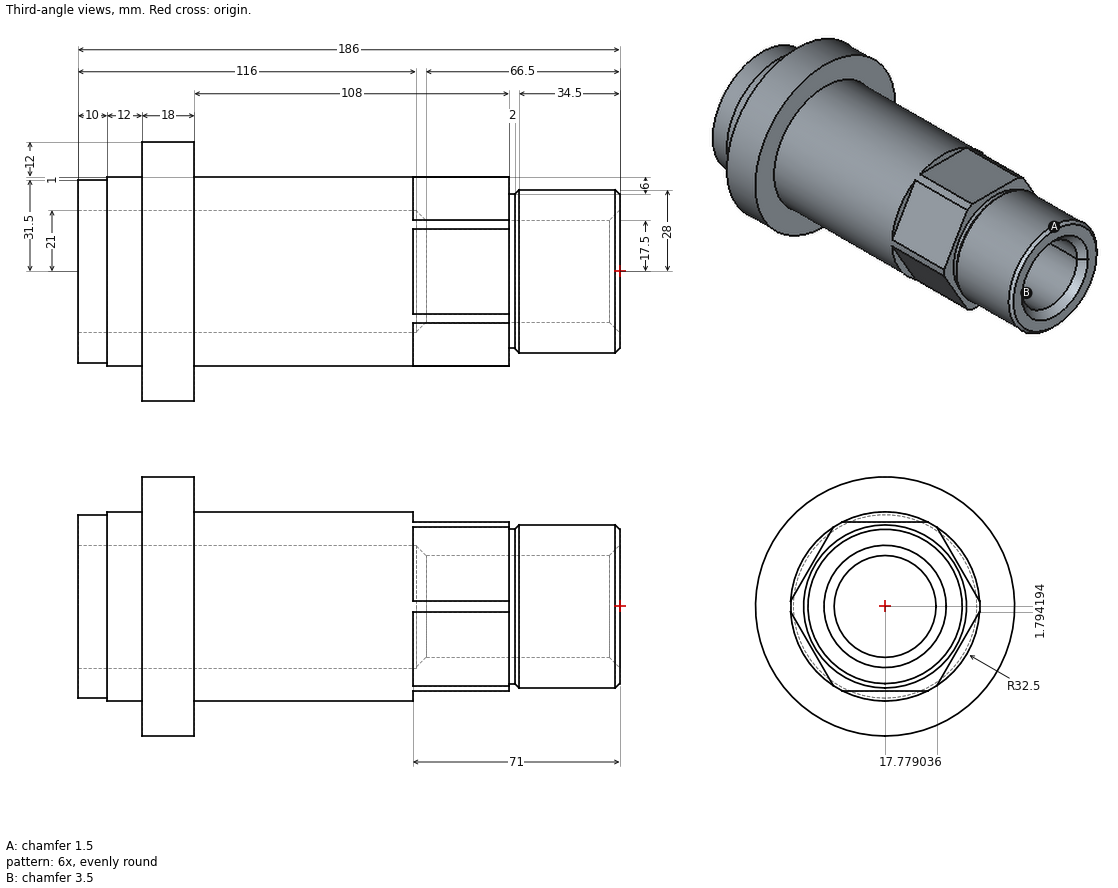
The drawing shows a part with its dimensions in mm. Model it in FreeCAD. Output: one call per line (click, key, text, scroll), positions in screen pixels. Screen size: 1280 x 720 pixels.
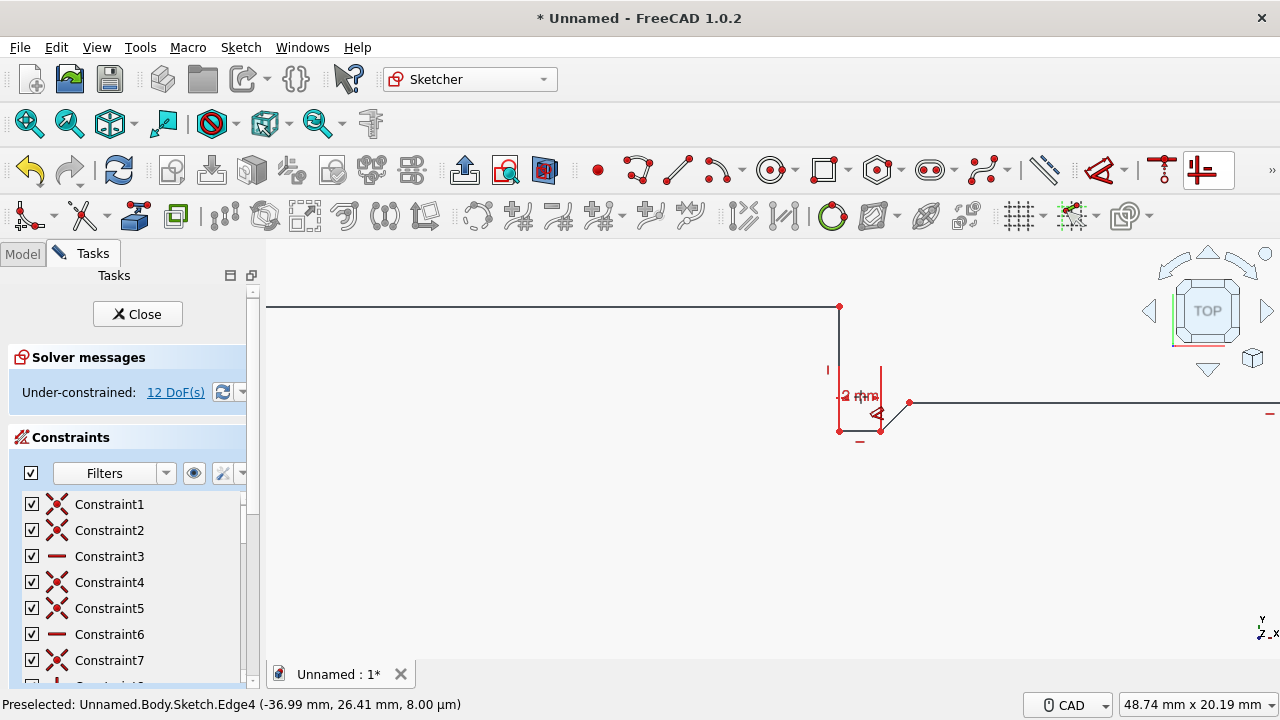
click(839, 394)
click(873, 369)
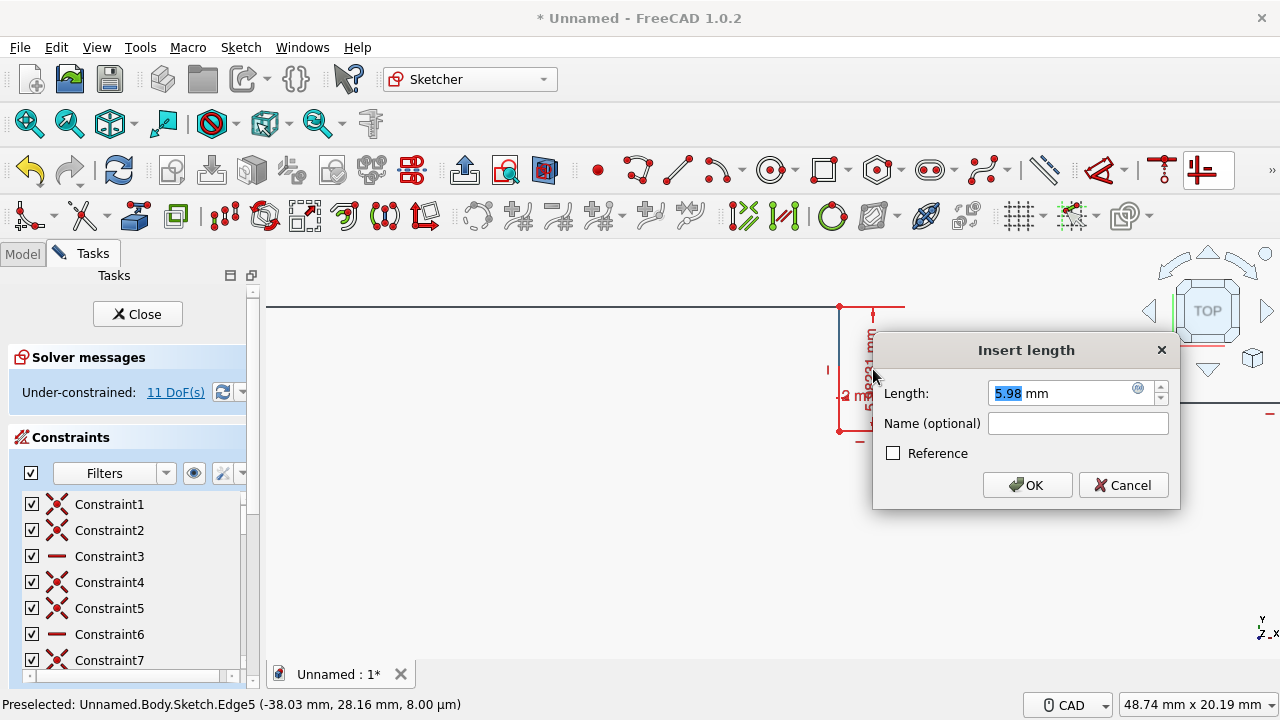
text(6)
key(Return)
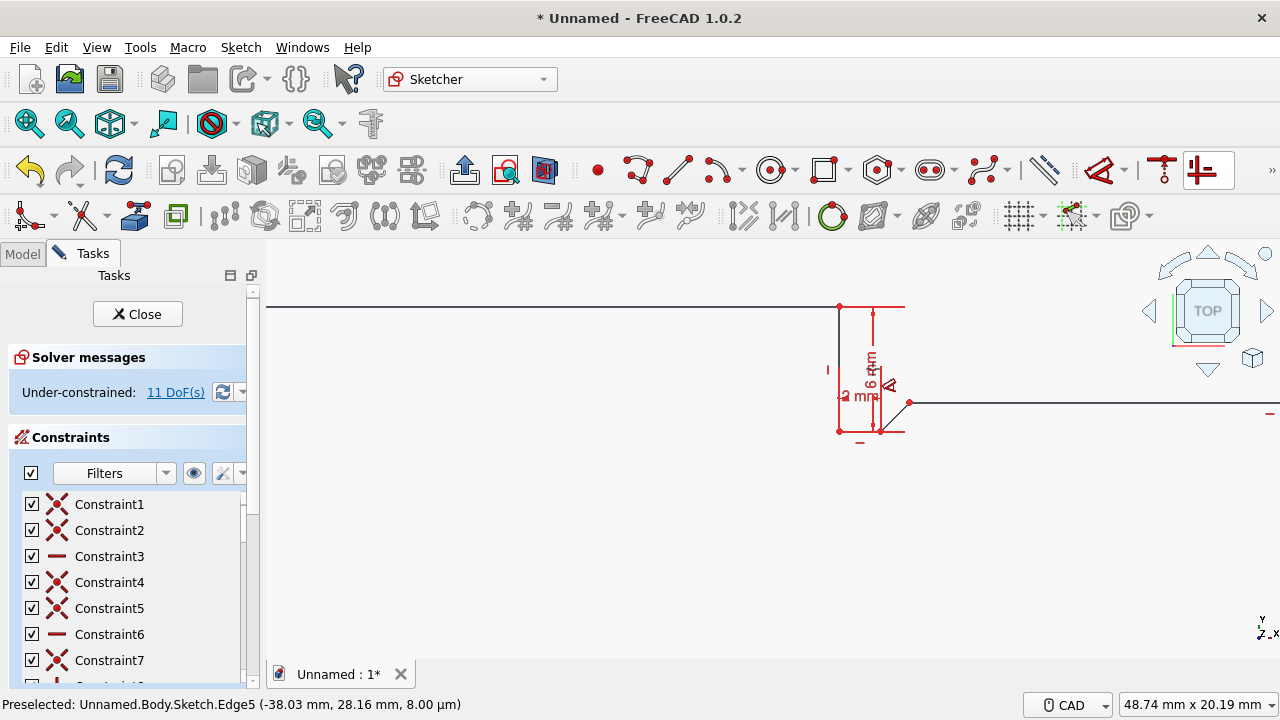
scroll(904, 435, down, 9)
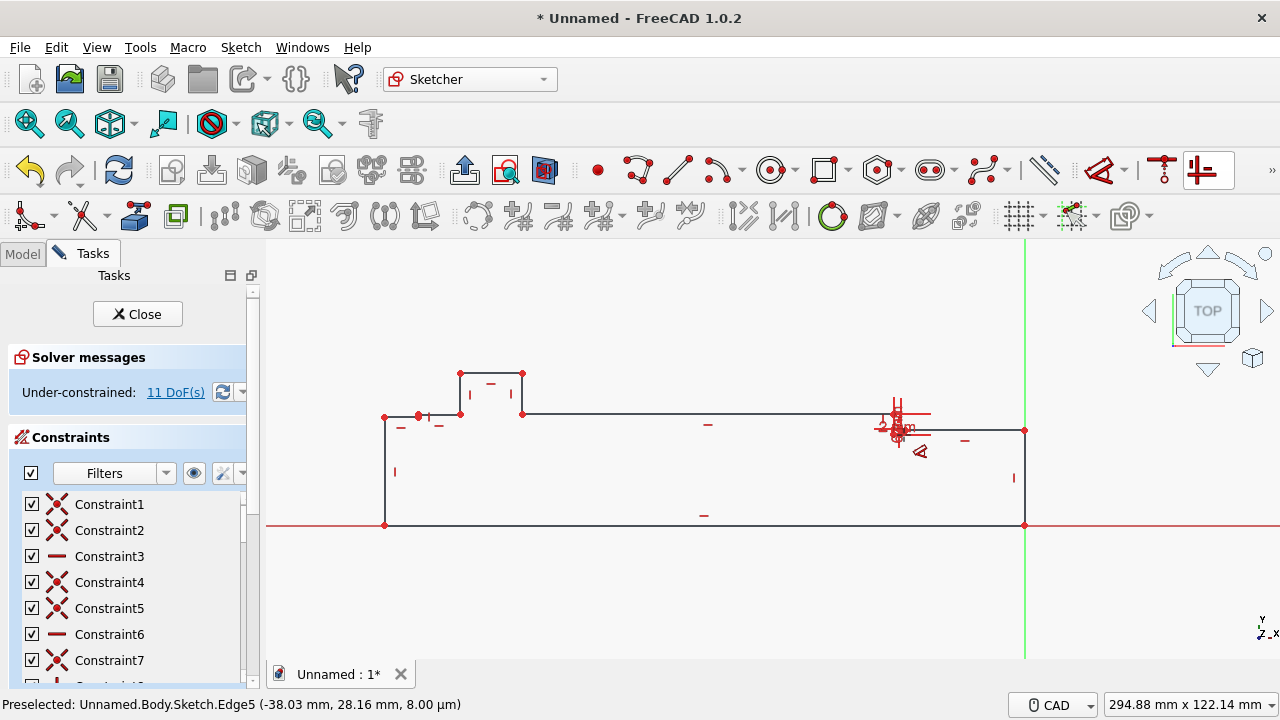
scroll(419, 416, up, 13)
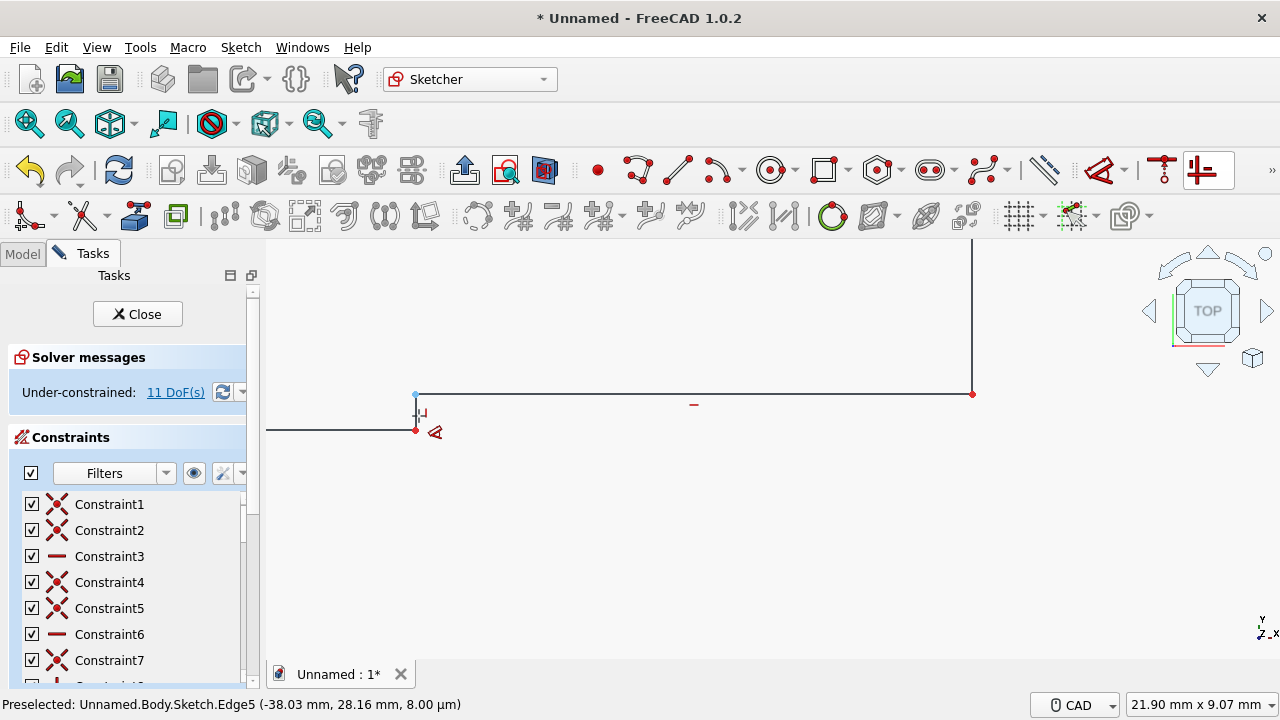
click(416, 412)
click(382, 412)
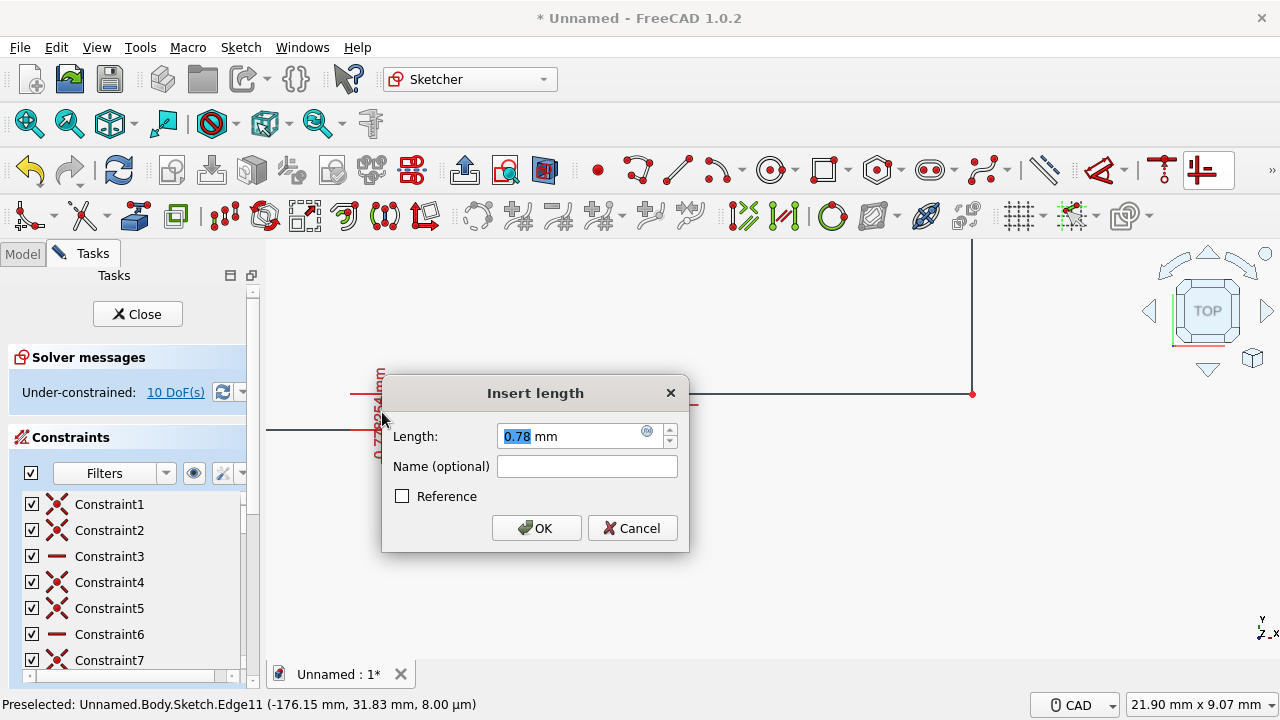
text(1)
key(Return)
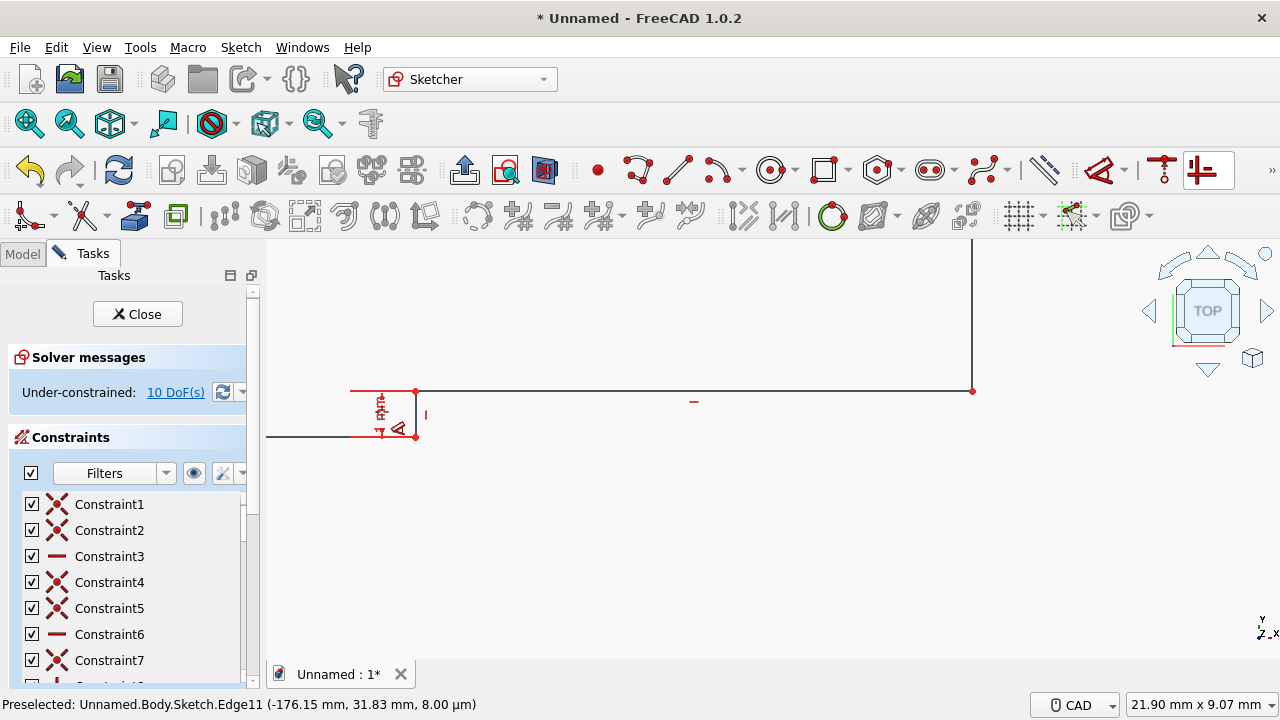
scroll(419, 416, down, 13)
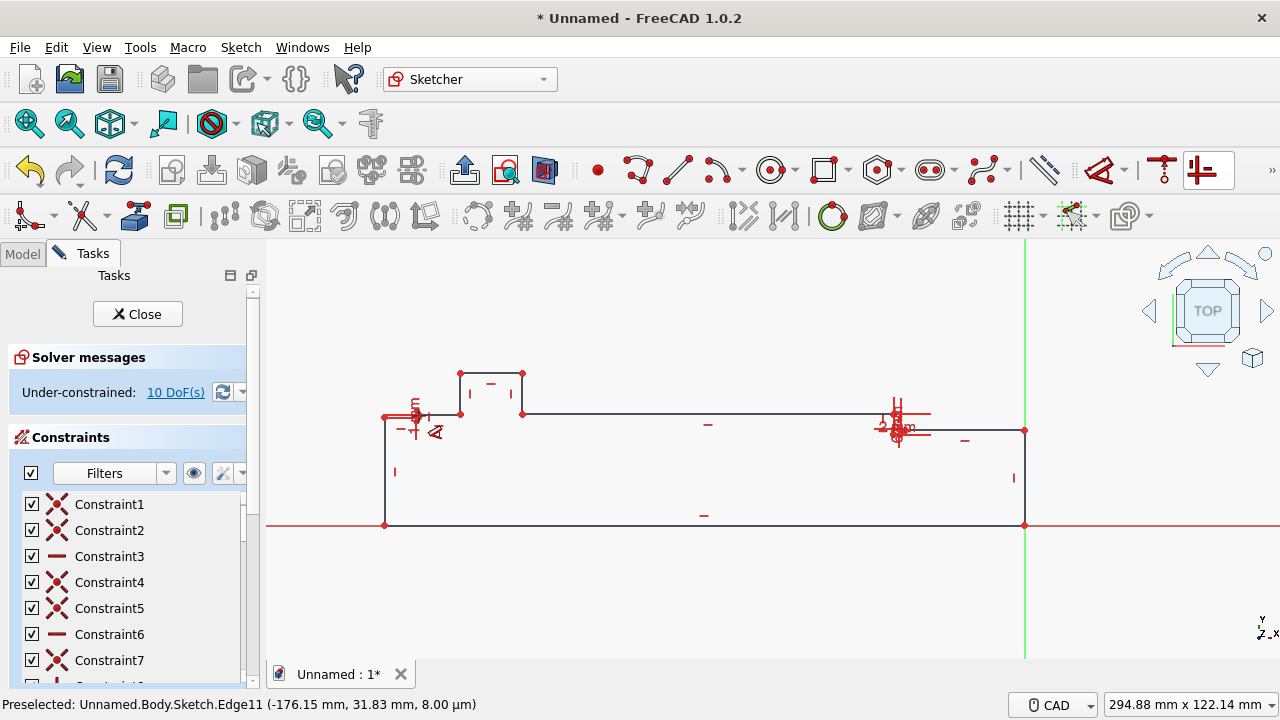
click(1025, 497)
click(1059, 478)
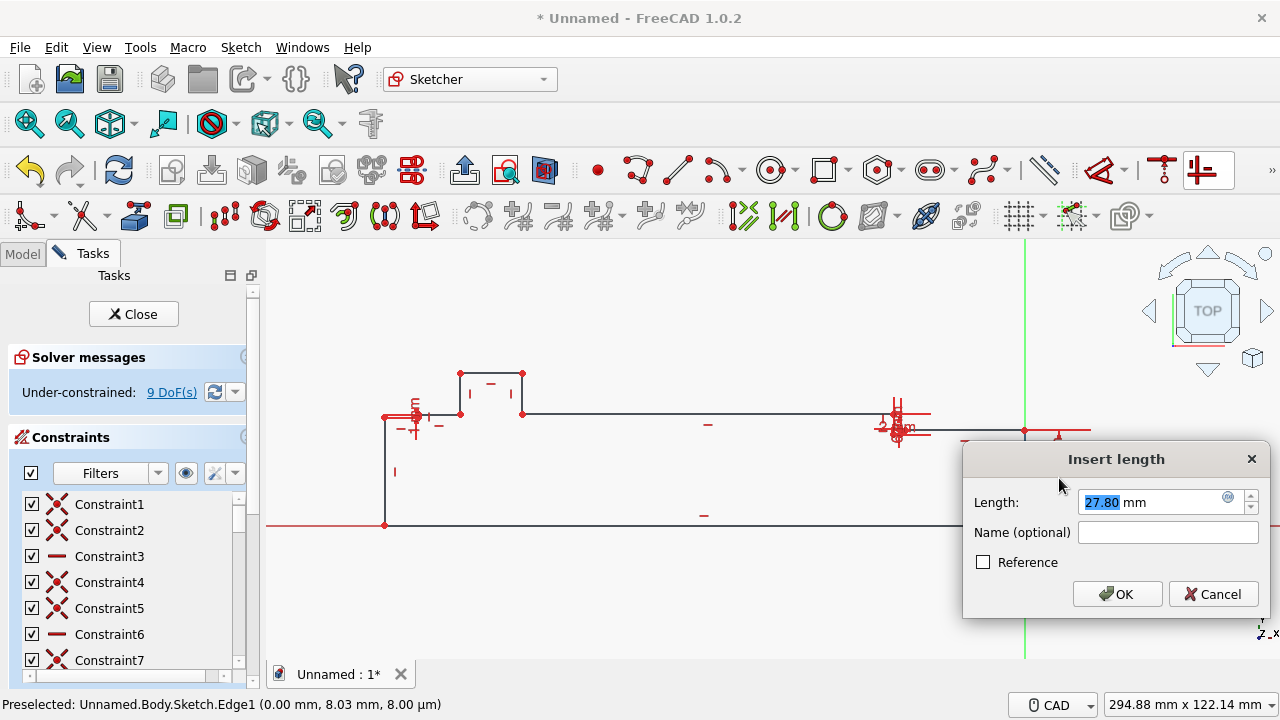
text(28)
key(Return)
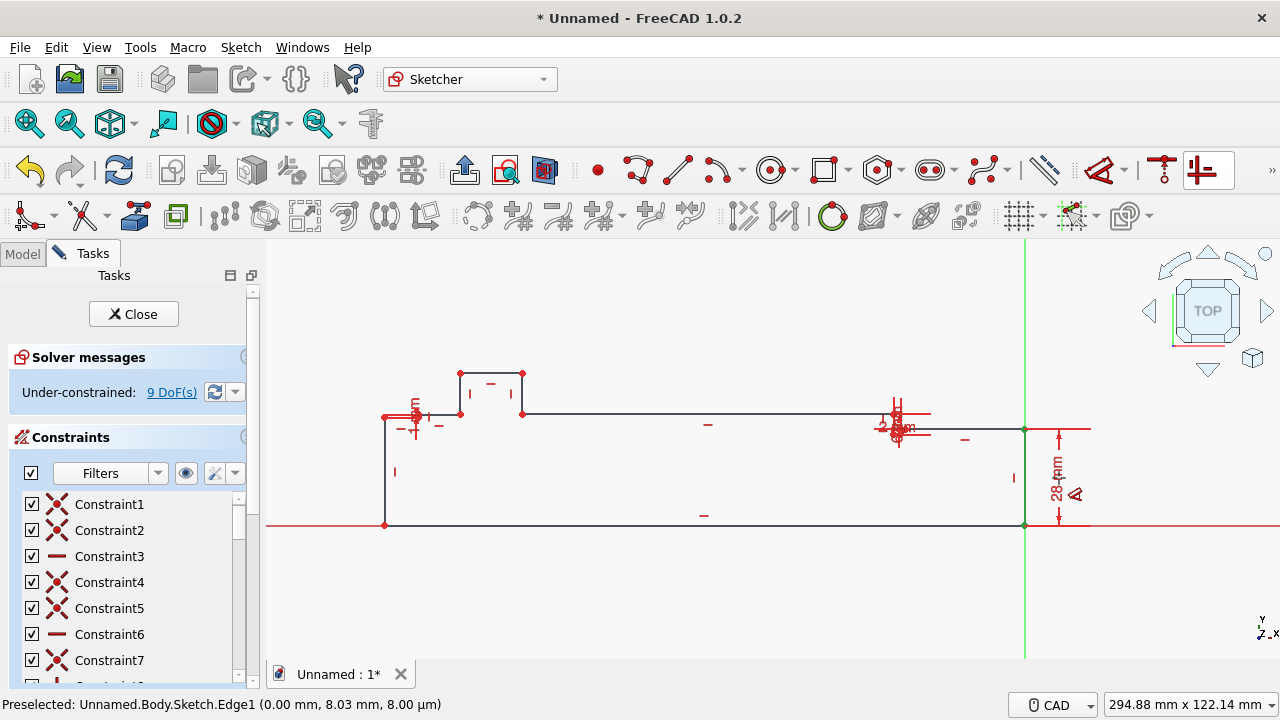
click(522, 402)
click(488, 394)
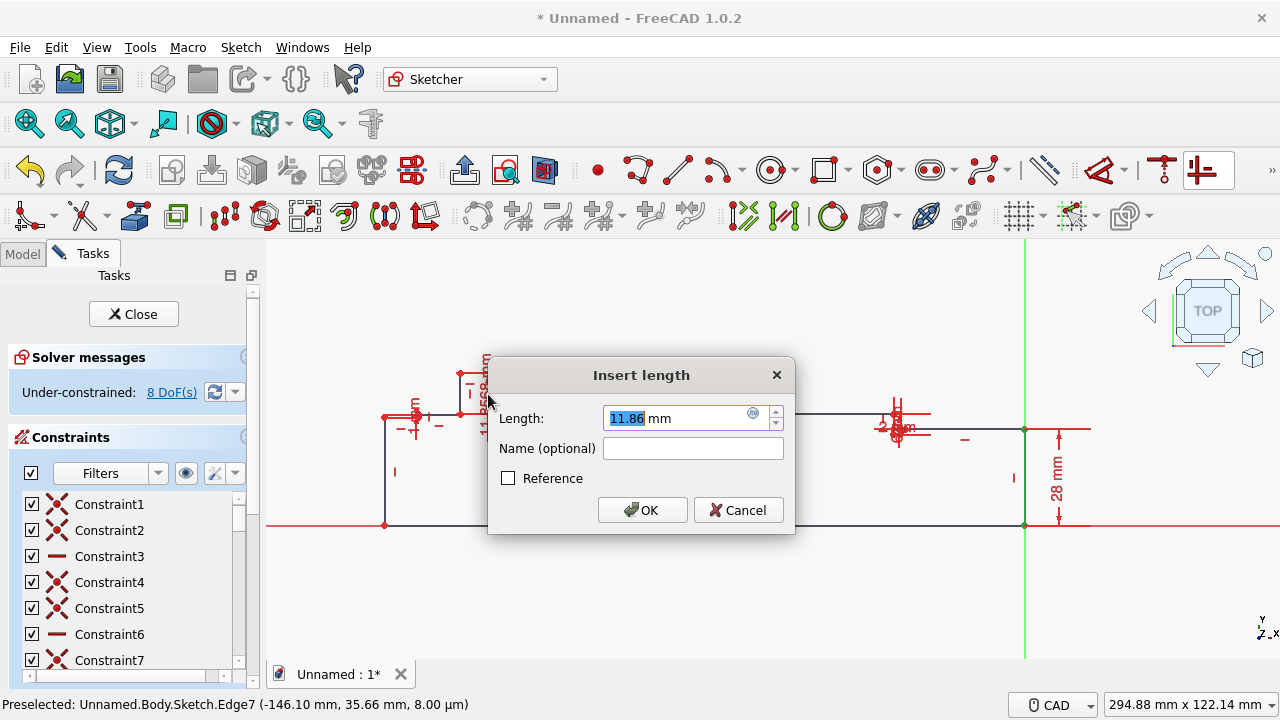
text(12)
key(Return)